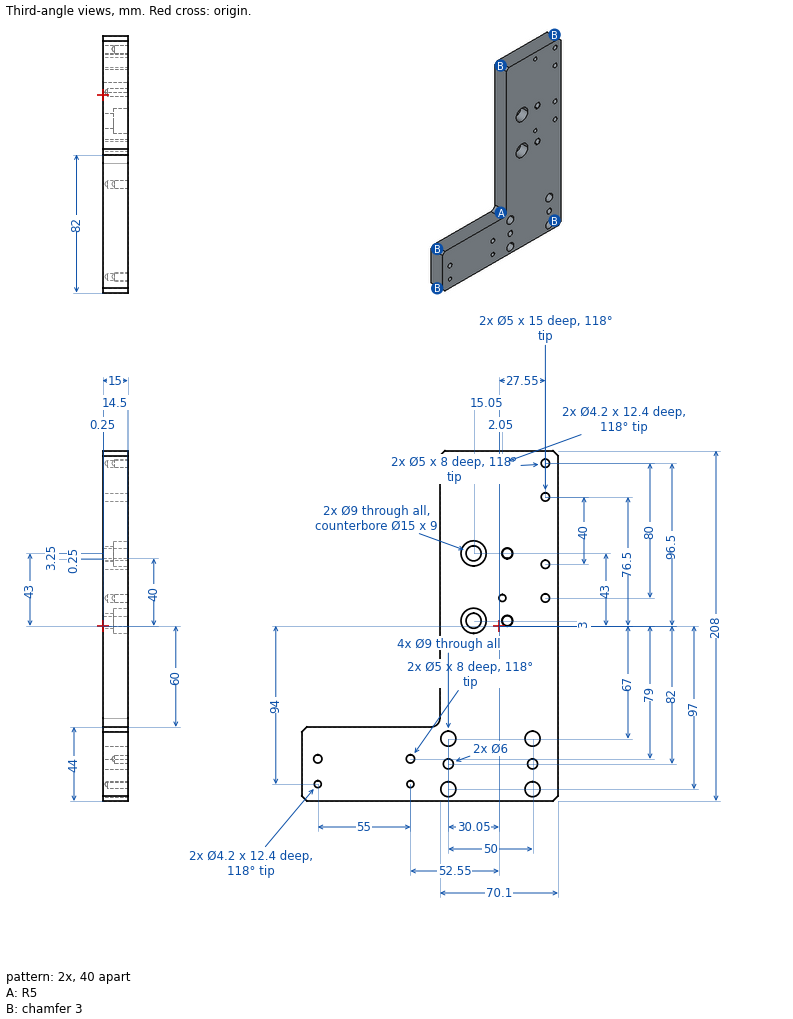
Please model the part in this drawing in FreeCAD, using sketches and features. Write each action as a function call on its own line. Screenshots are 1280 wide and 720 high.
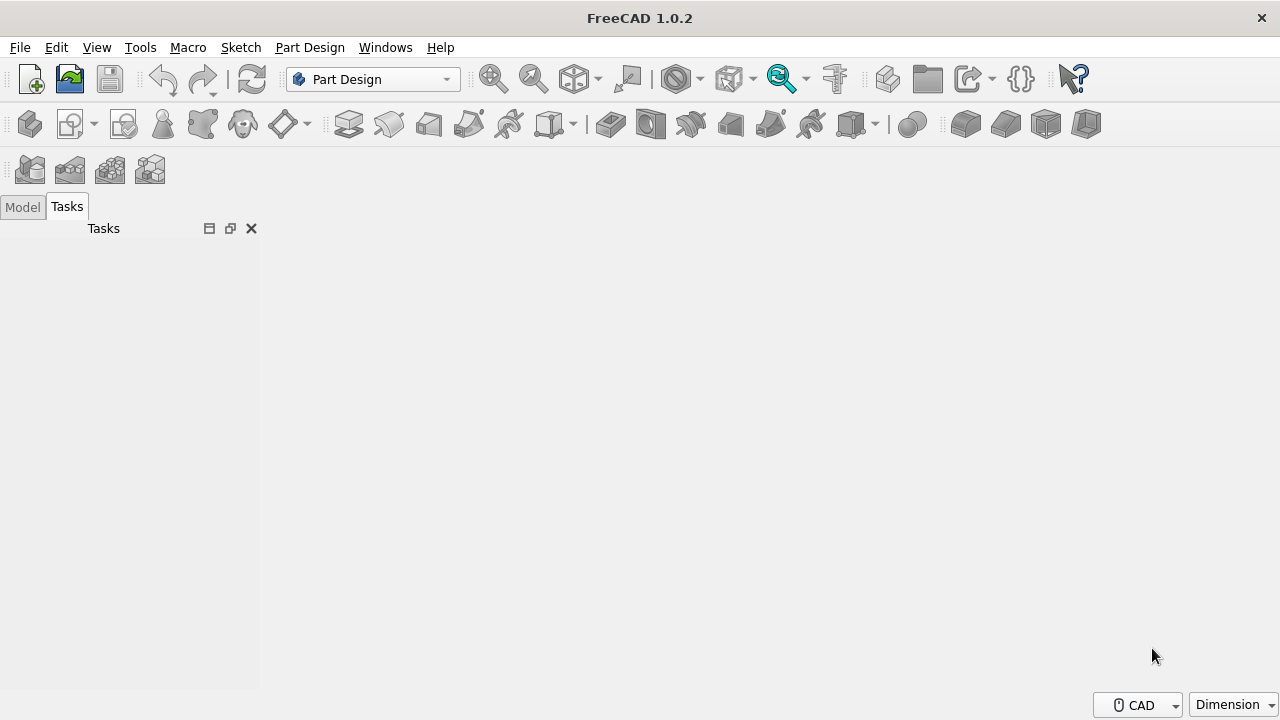
click(30, 80)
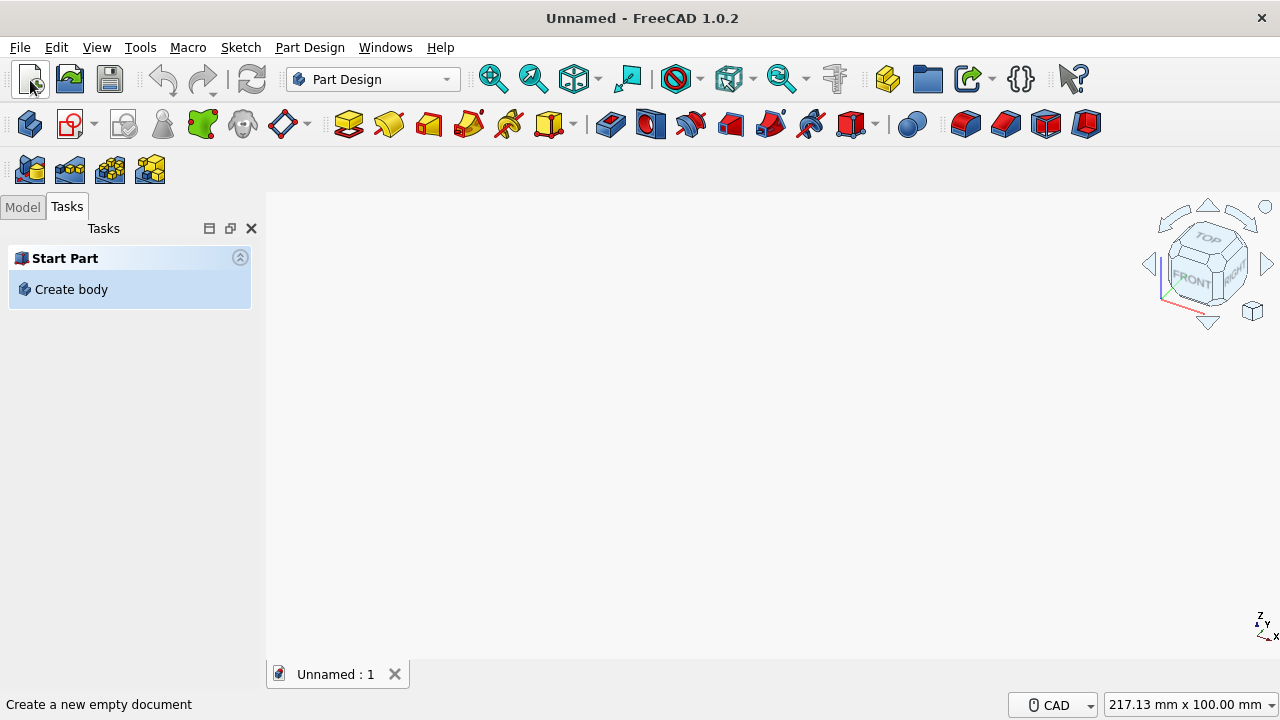
click(70, 124)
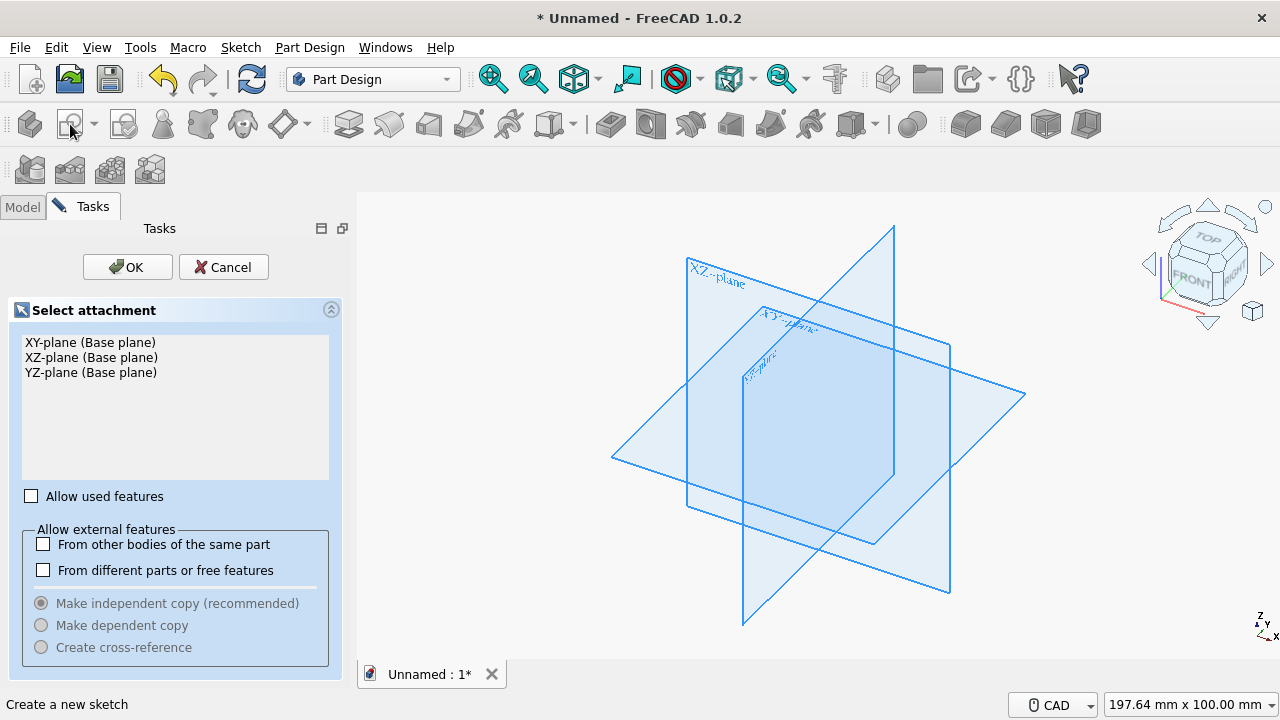
click(82, 372)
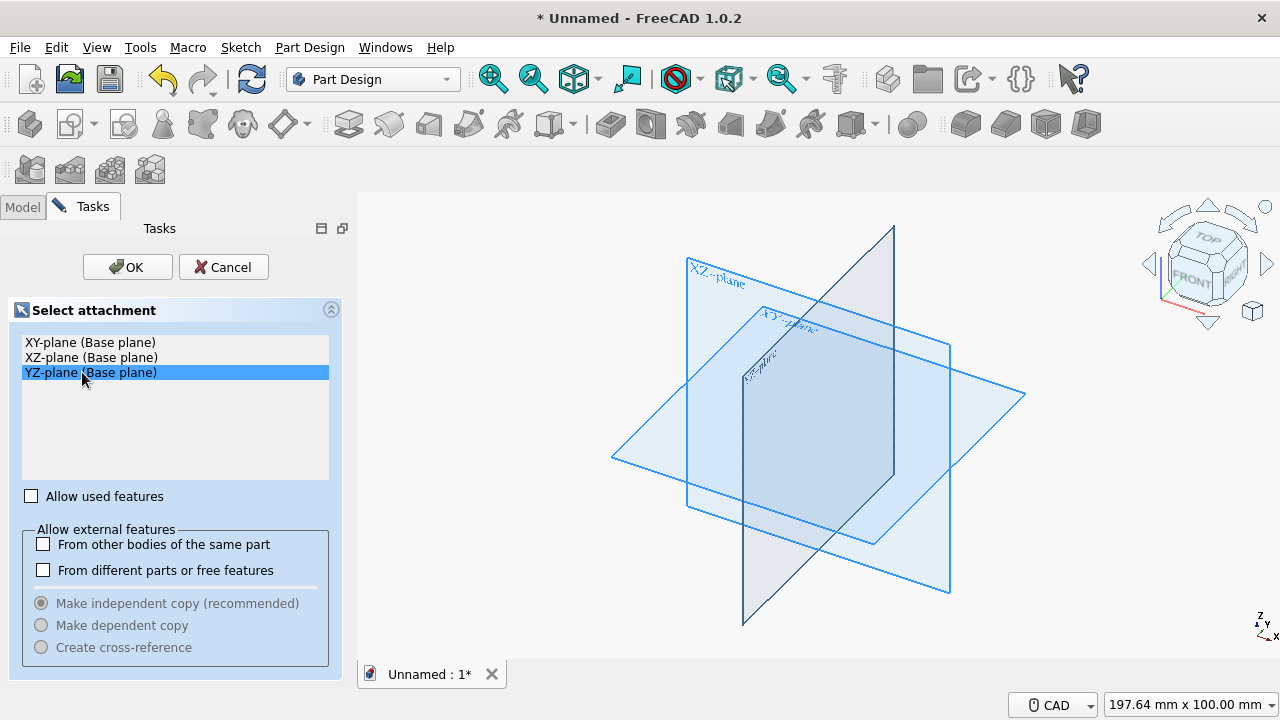
click(128, 267)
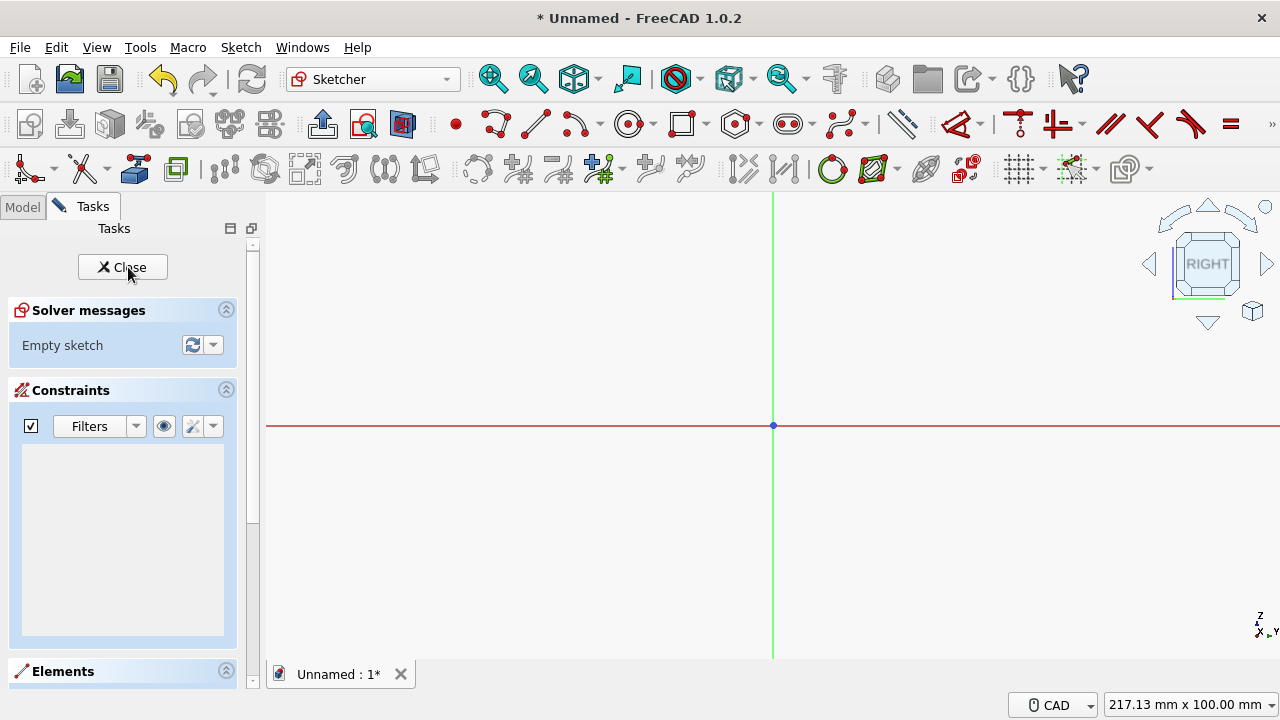
scroll(675, 426, down, 6)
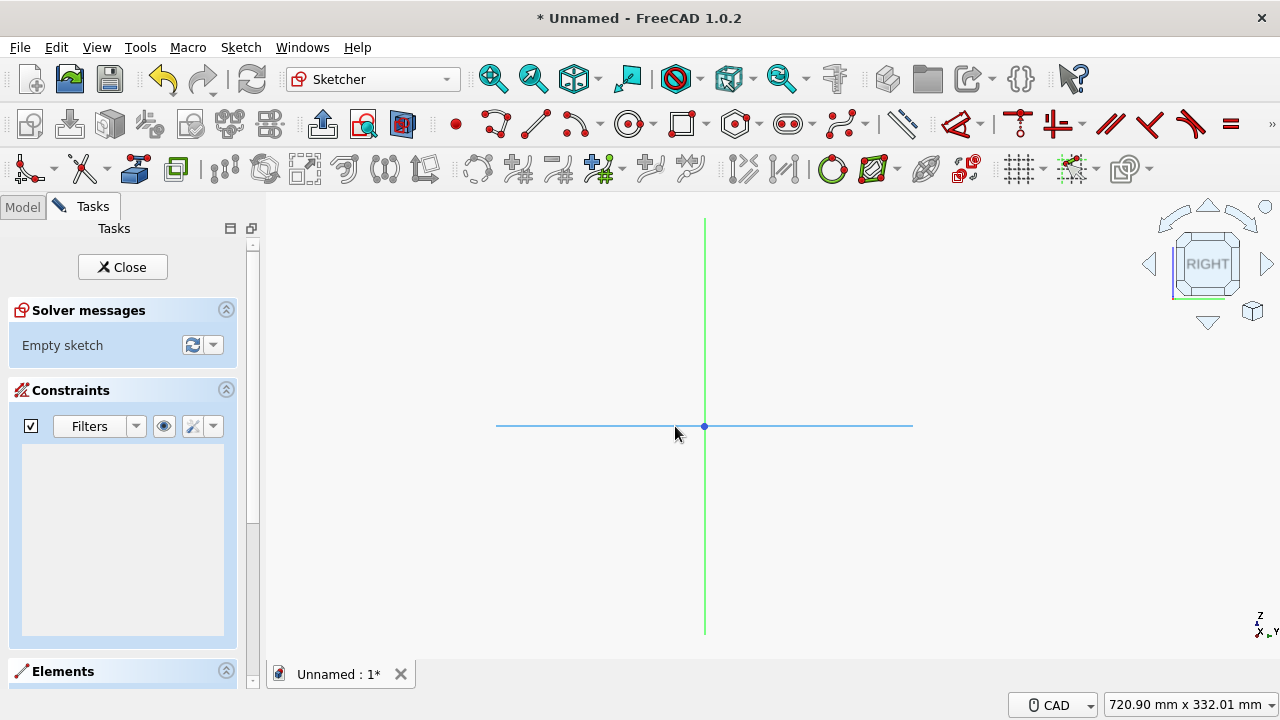
key(g)
key(v)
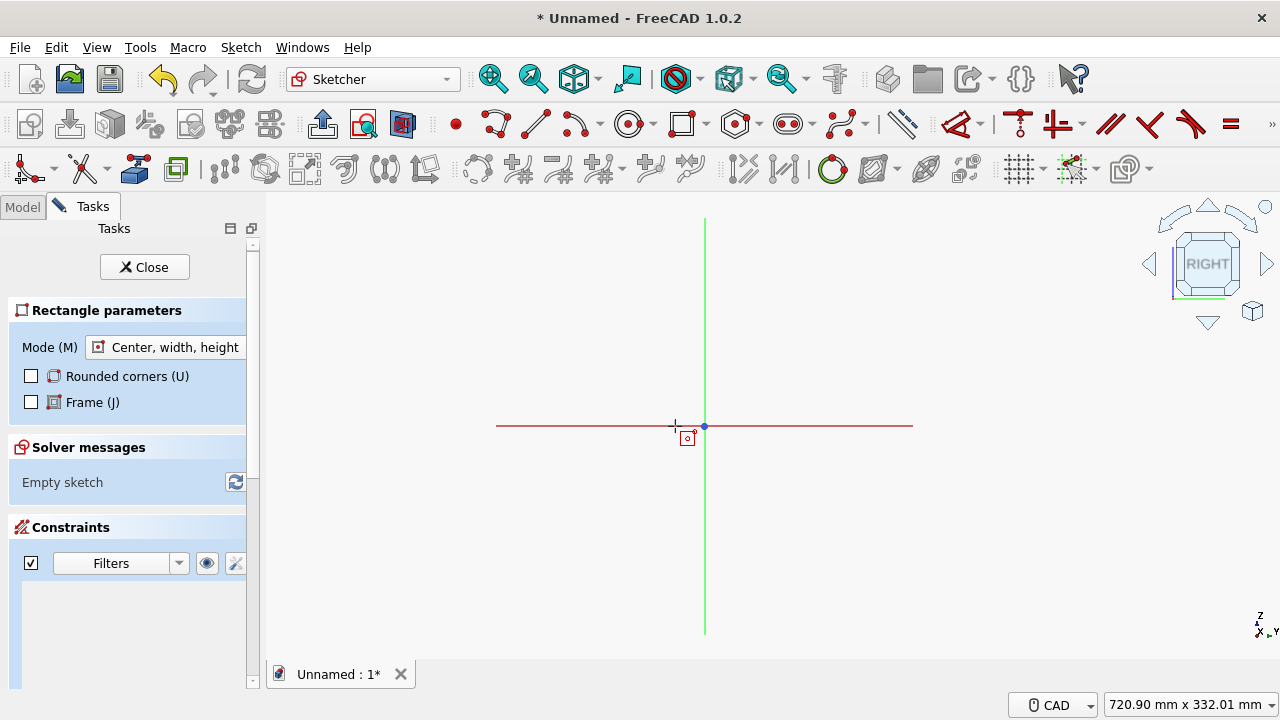
click(705, 426)
click(754, 280)
key(Escape)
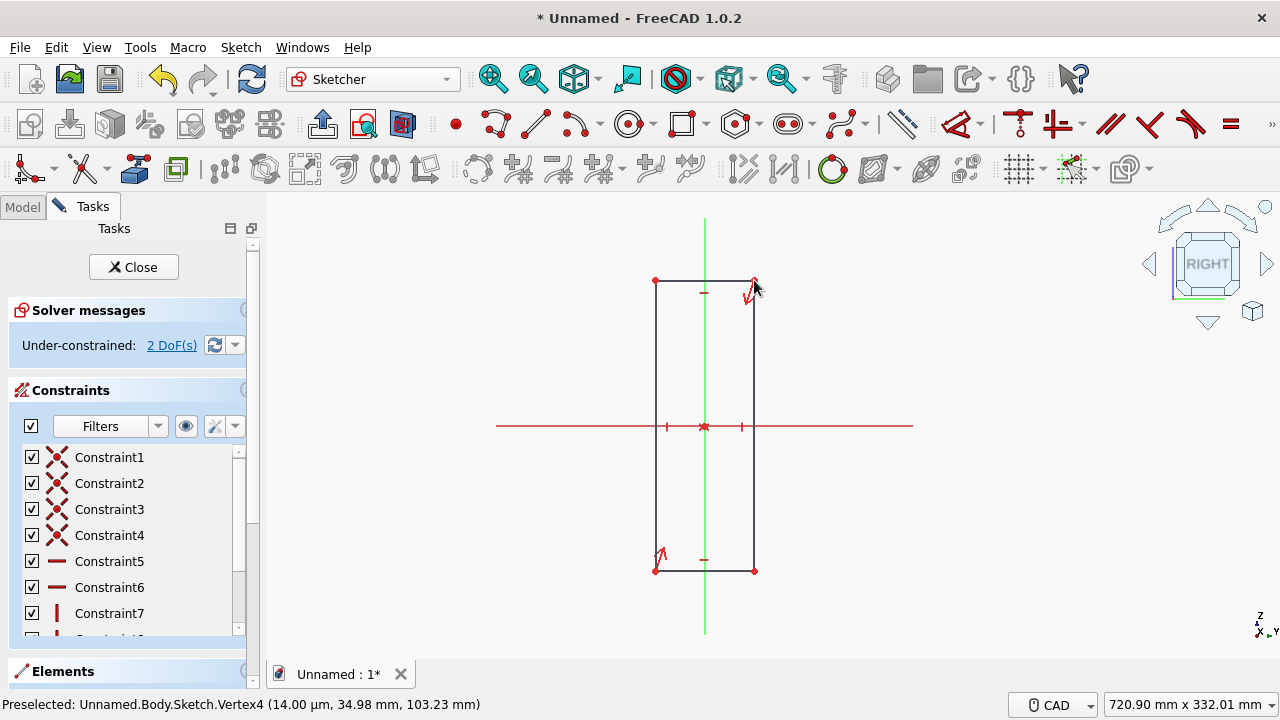
click(956, 124)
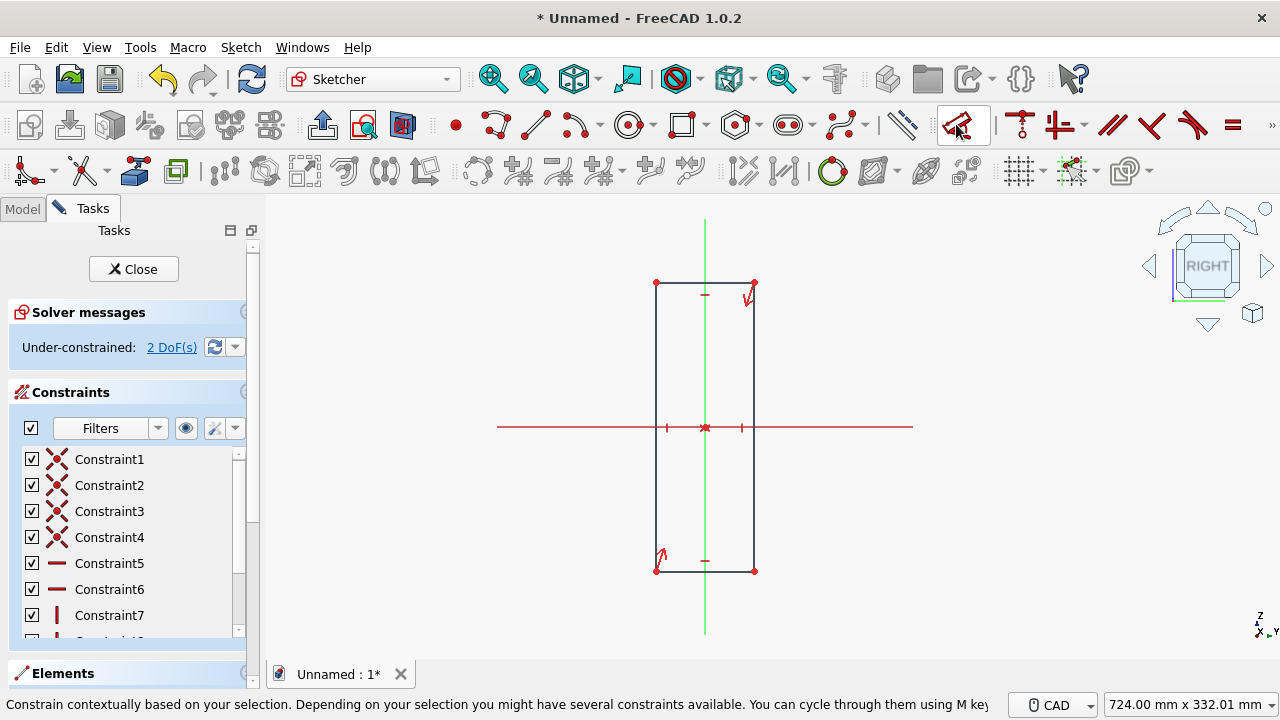
click(754, 485)
click(788, 361)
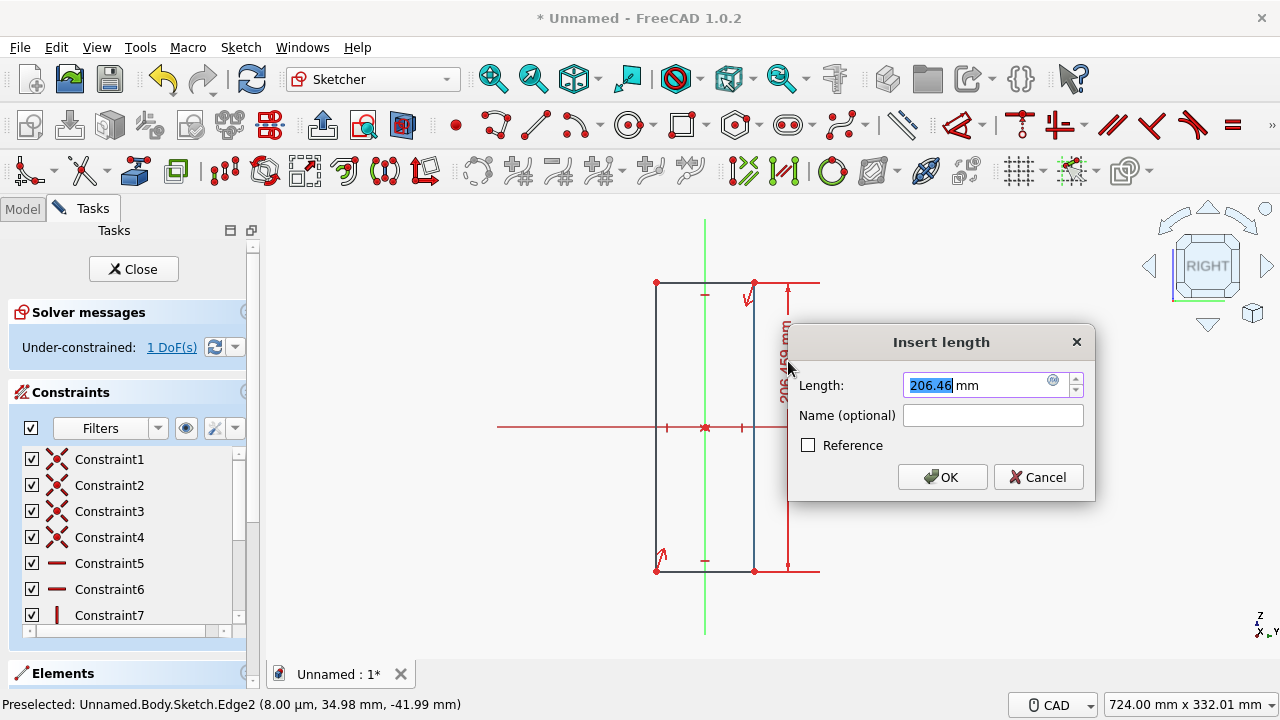
text(208)
key(Return)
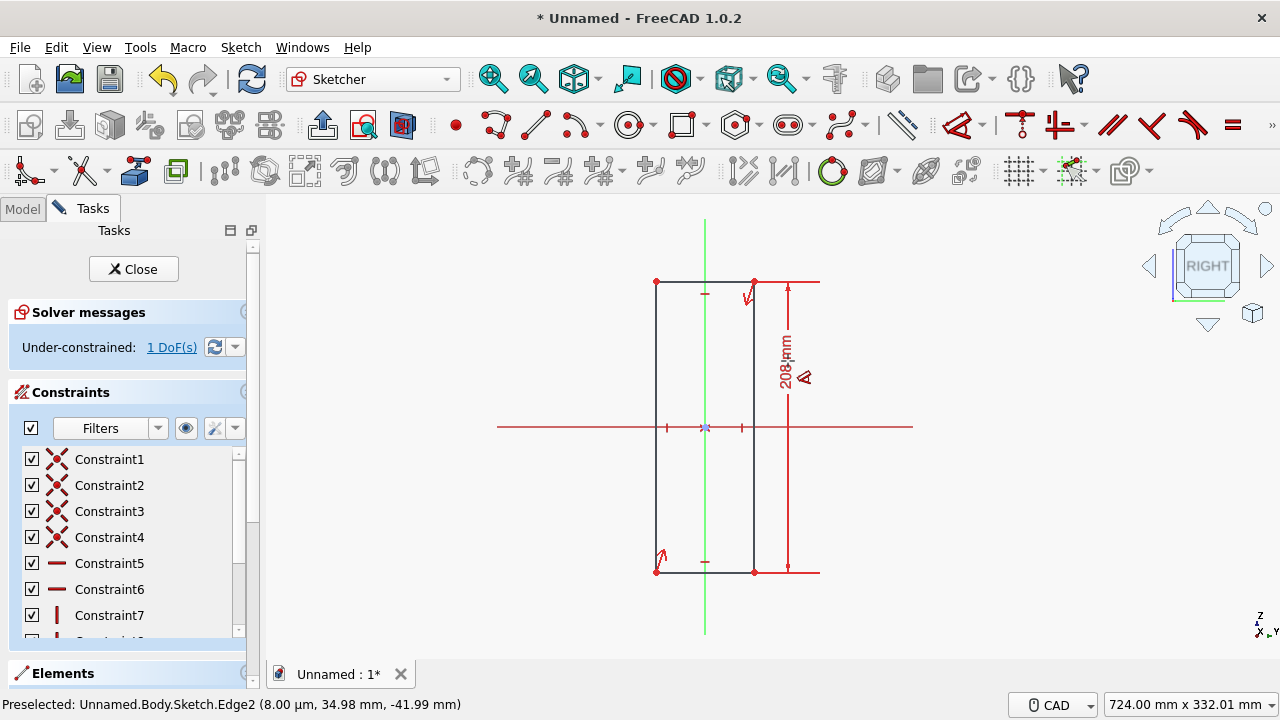
click(685, 573)
click(683, 607)